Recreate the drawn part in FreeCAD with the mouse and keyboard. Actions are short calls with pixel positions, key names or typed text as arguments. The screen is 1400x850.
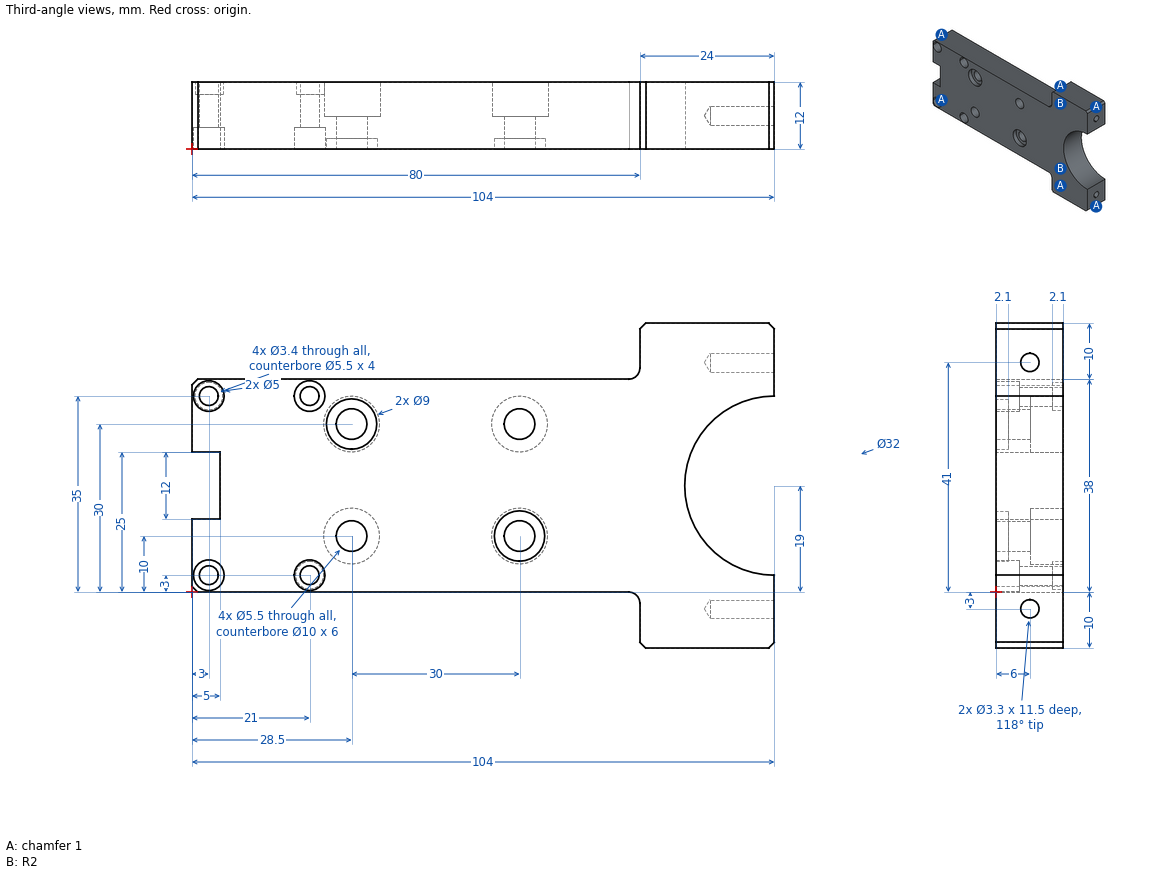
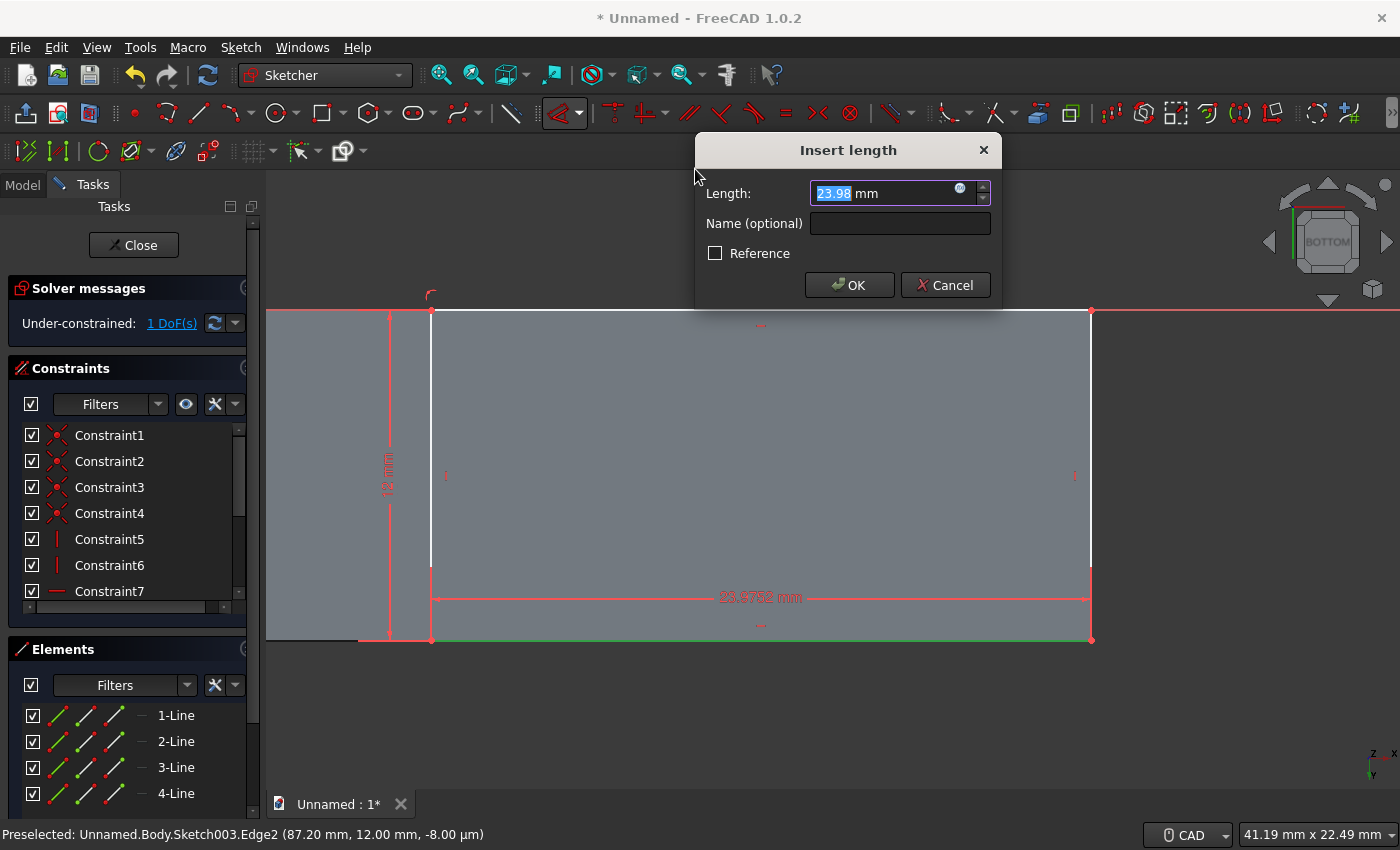
text(24)
key(Return)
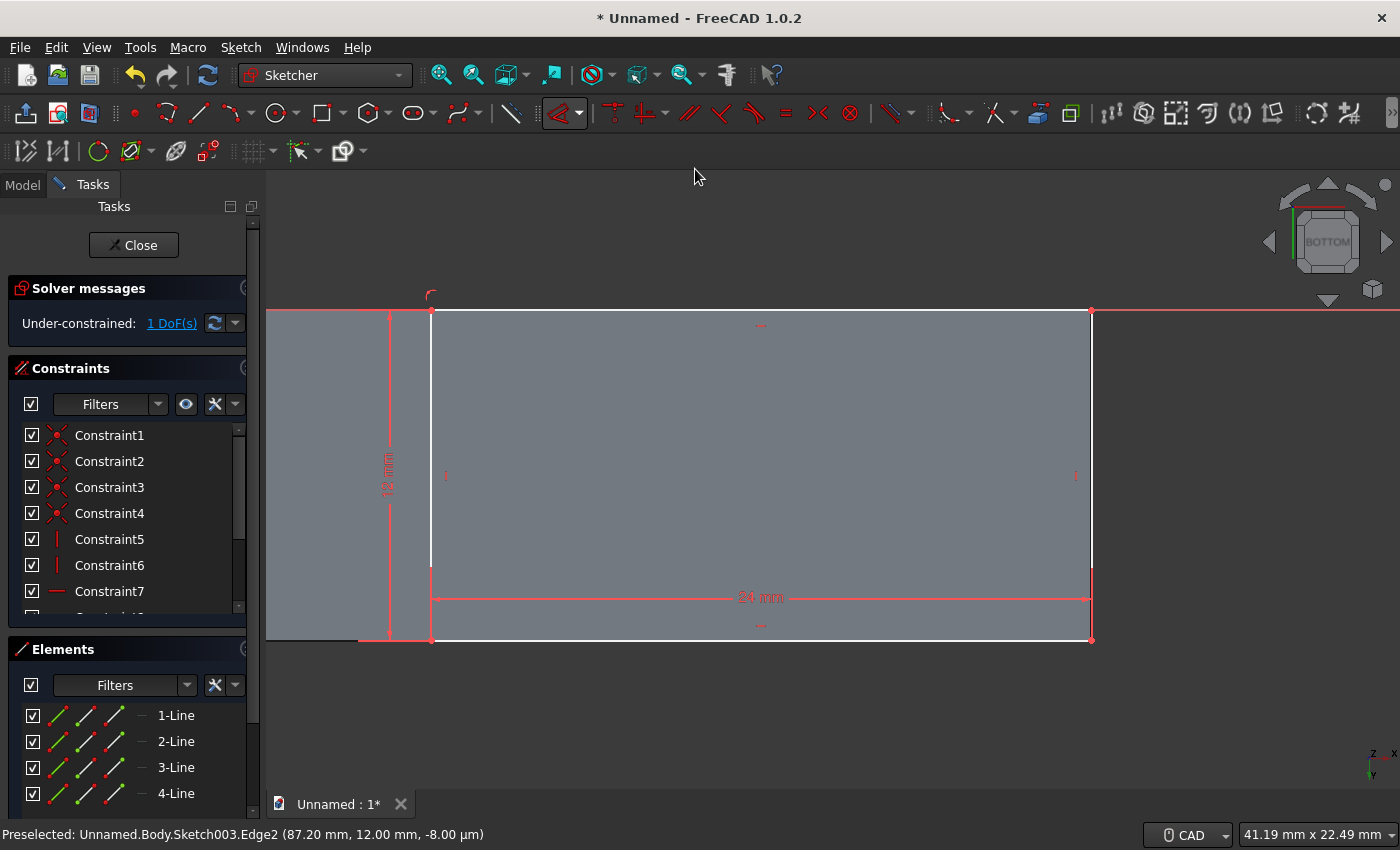
click(431, 310)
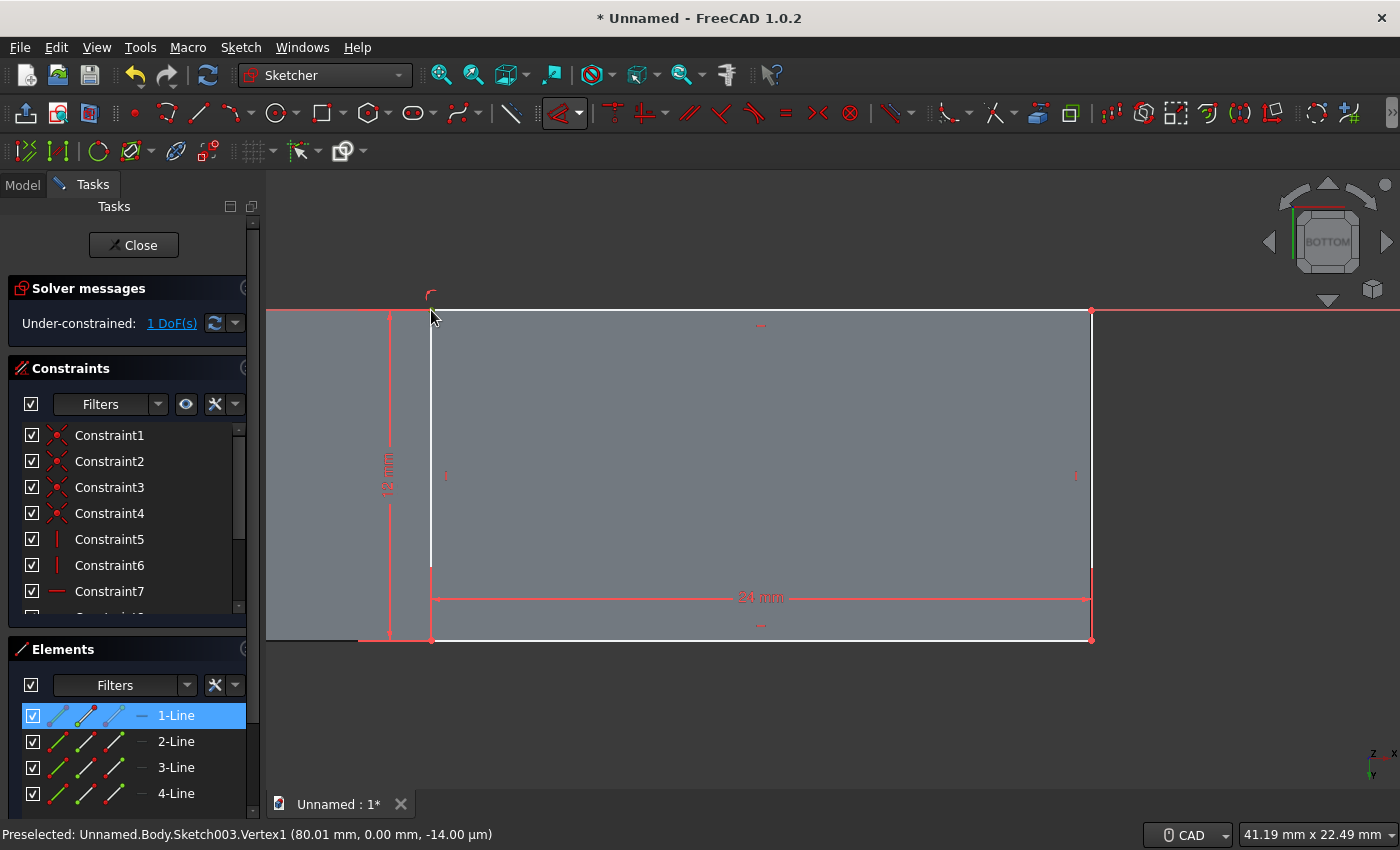
click(582, 114)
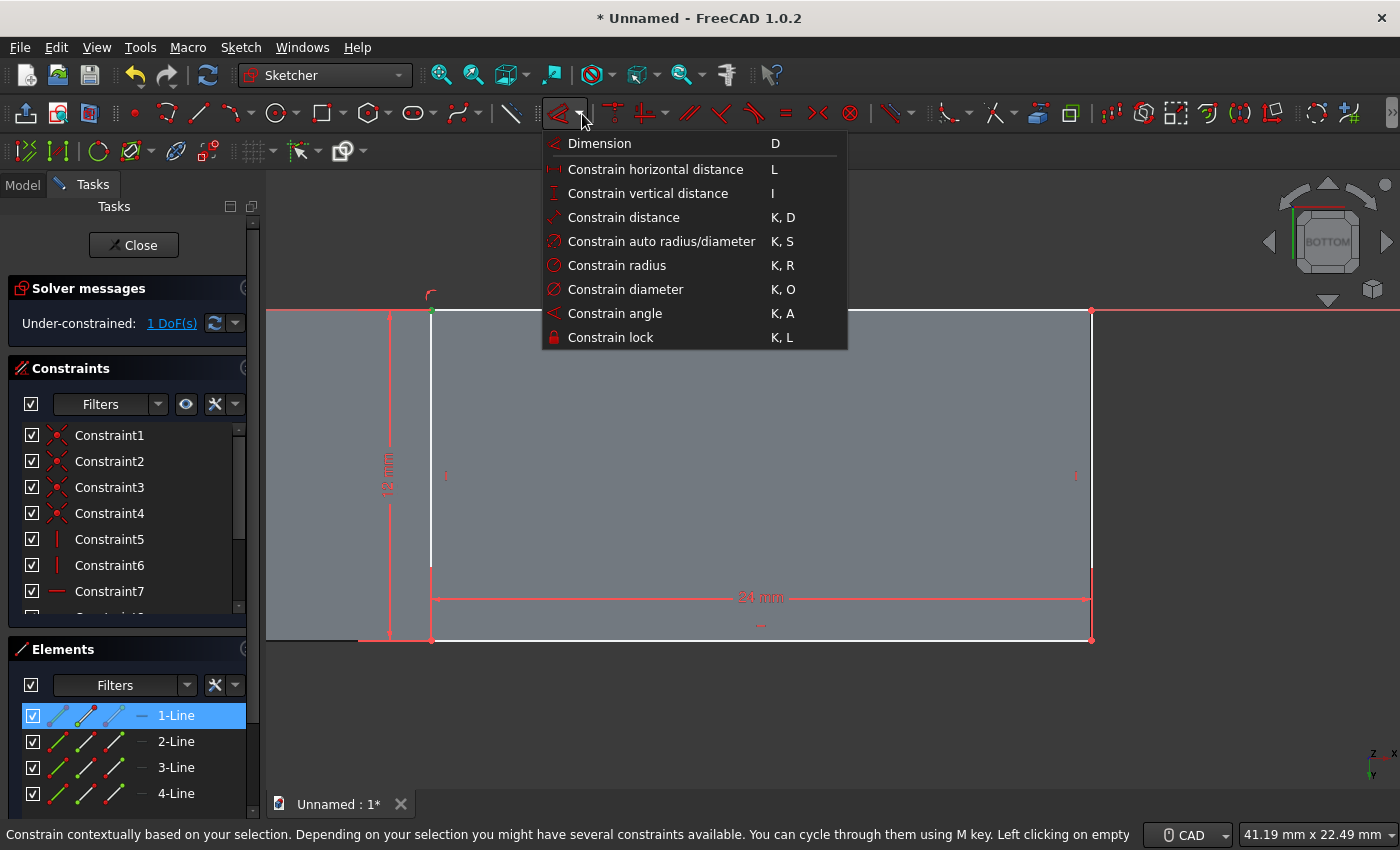
click(695, 169)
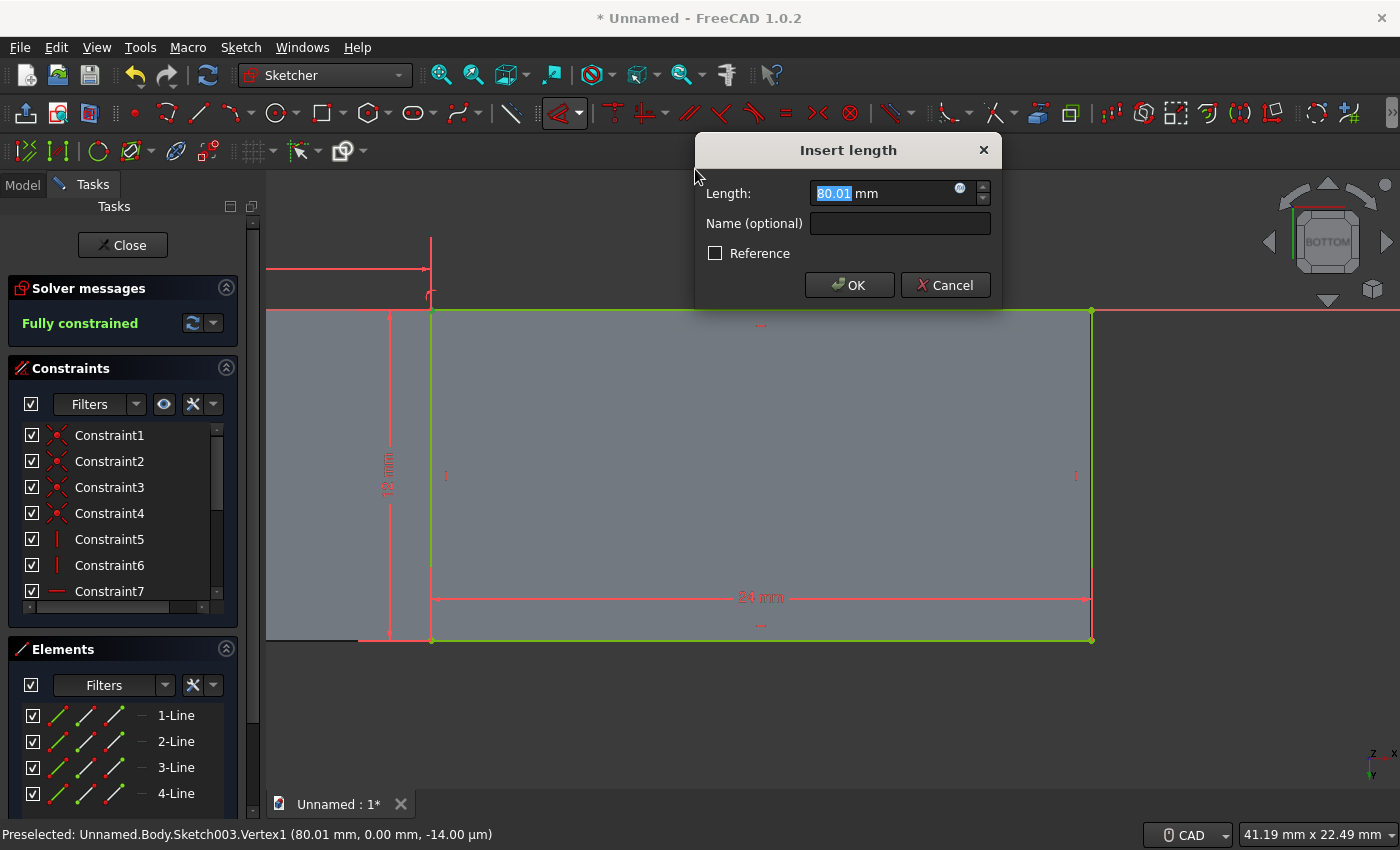
text(80)
key(Return)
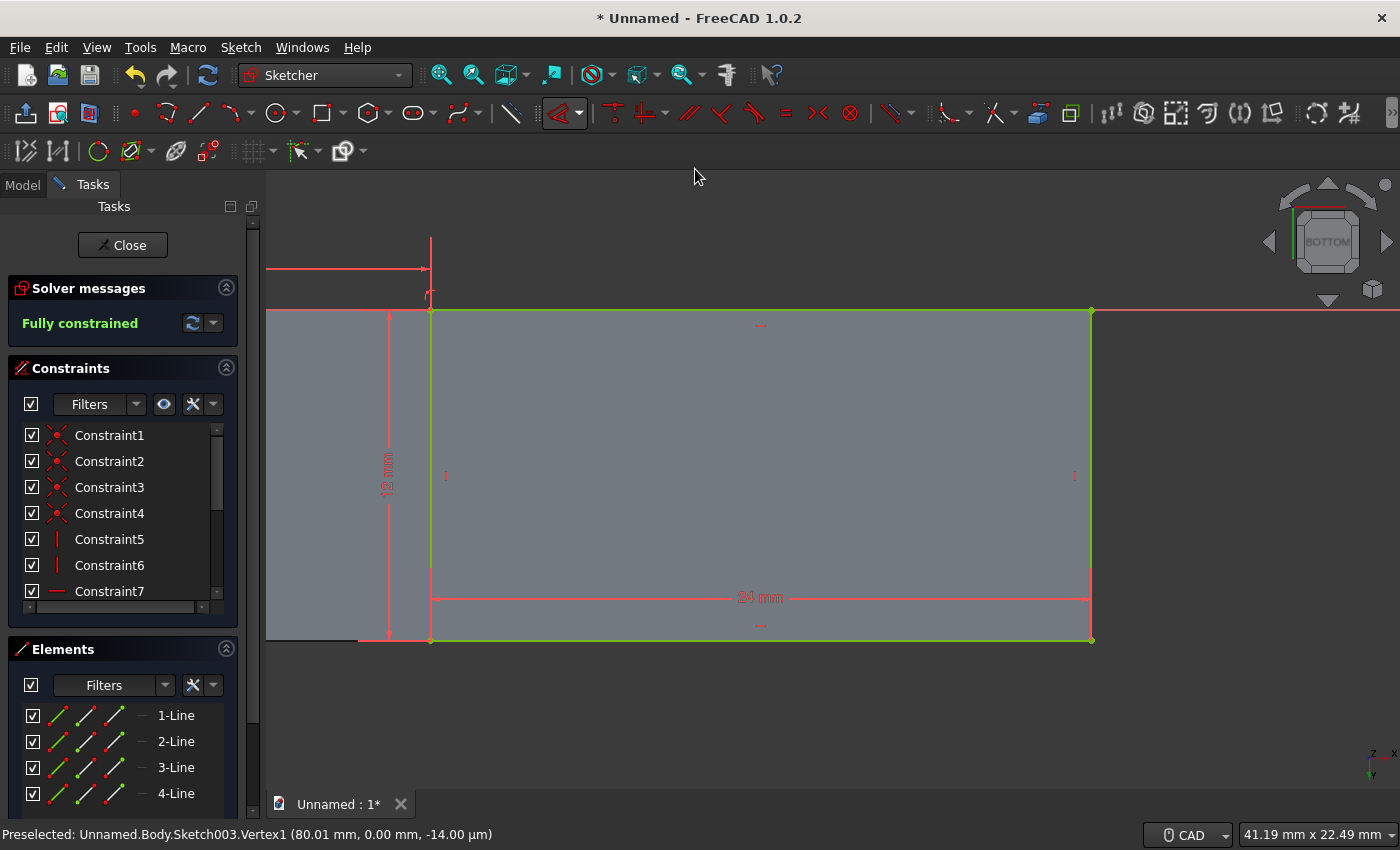
click(123, 245)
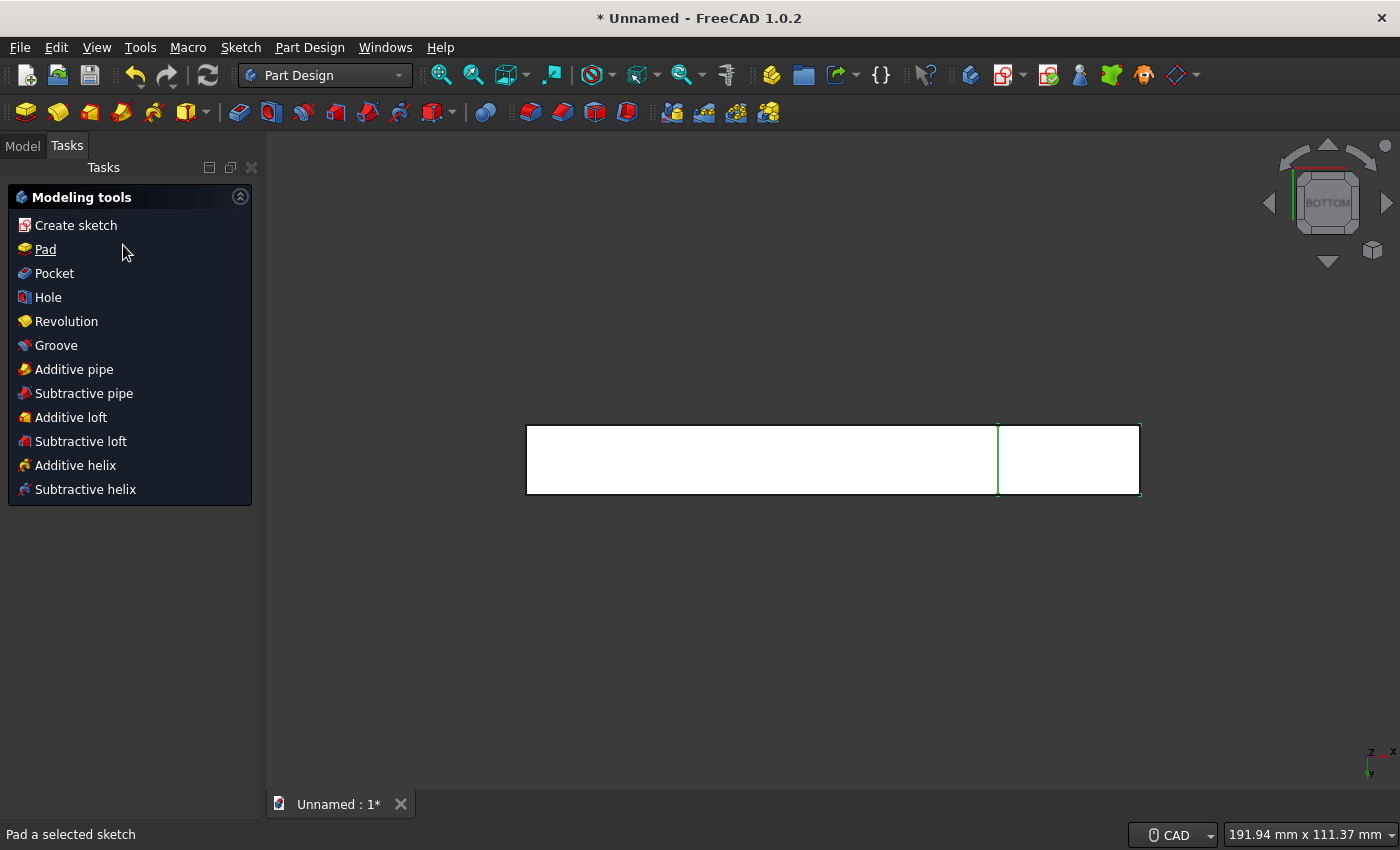
click(26, 112)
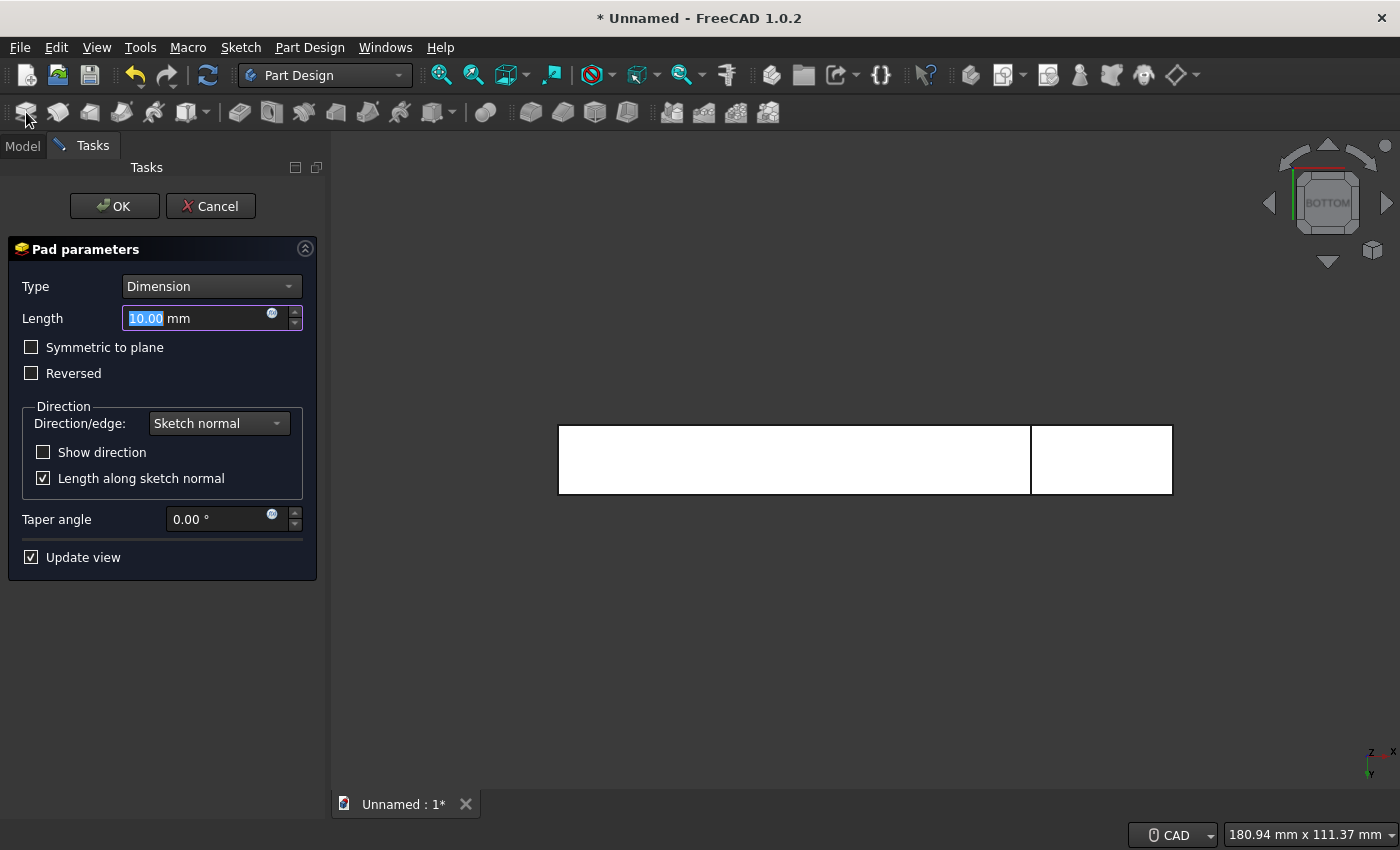
text(10)
key(Tab)